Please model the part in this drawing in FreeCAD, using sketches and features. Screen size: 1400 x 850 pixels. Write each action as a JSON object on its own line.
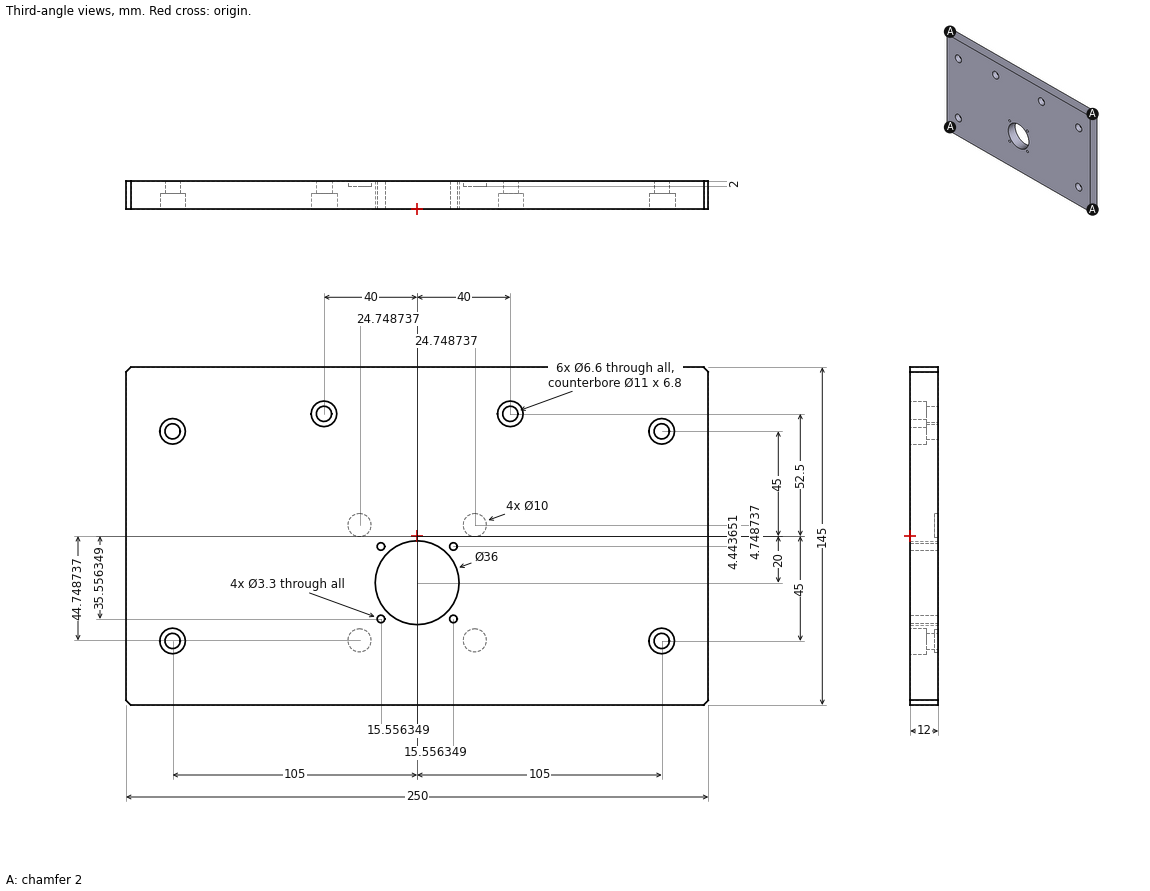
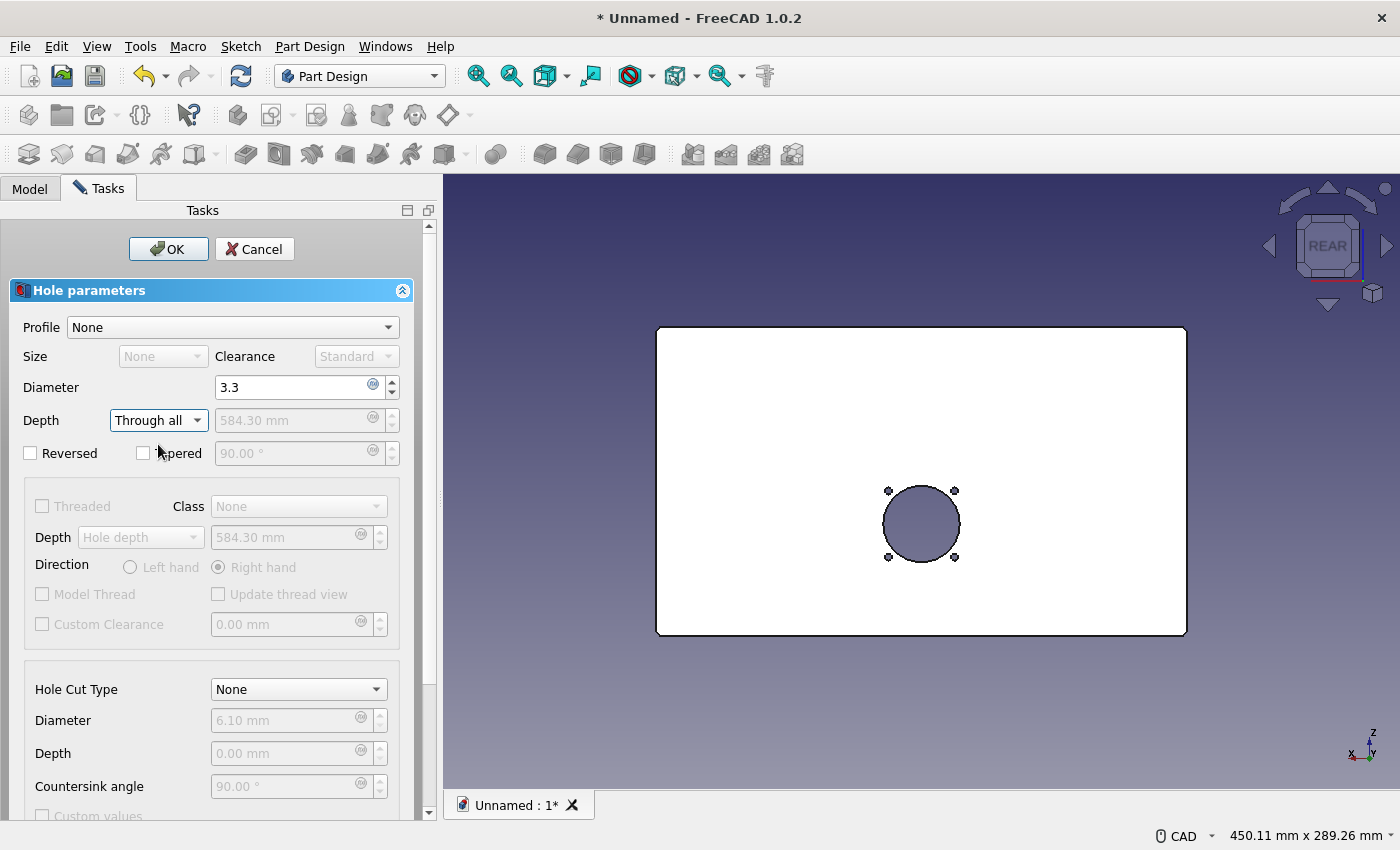
{"action": "left_click", "coordinate": [169, 249]}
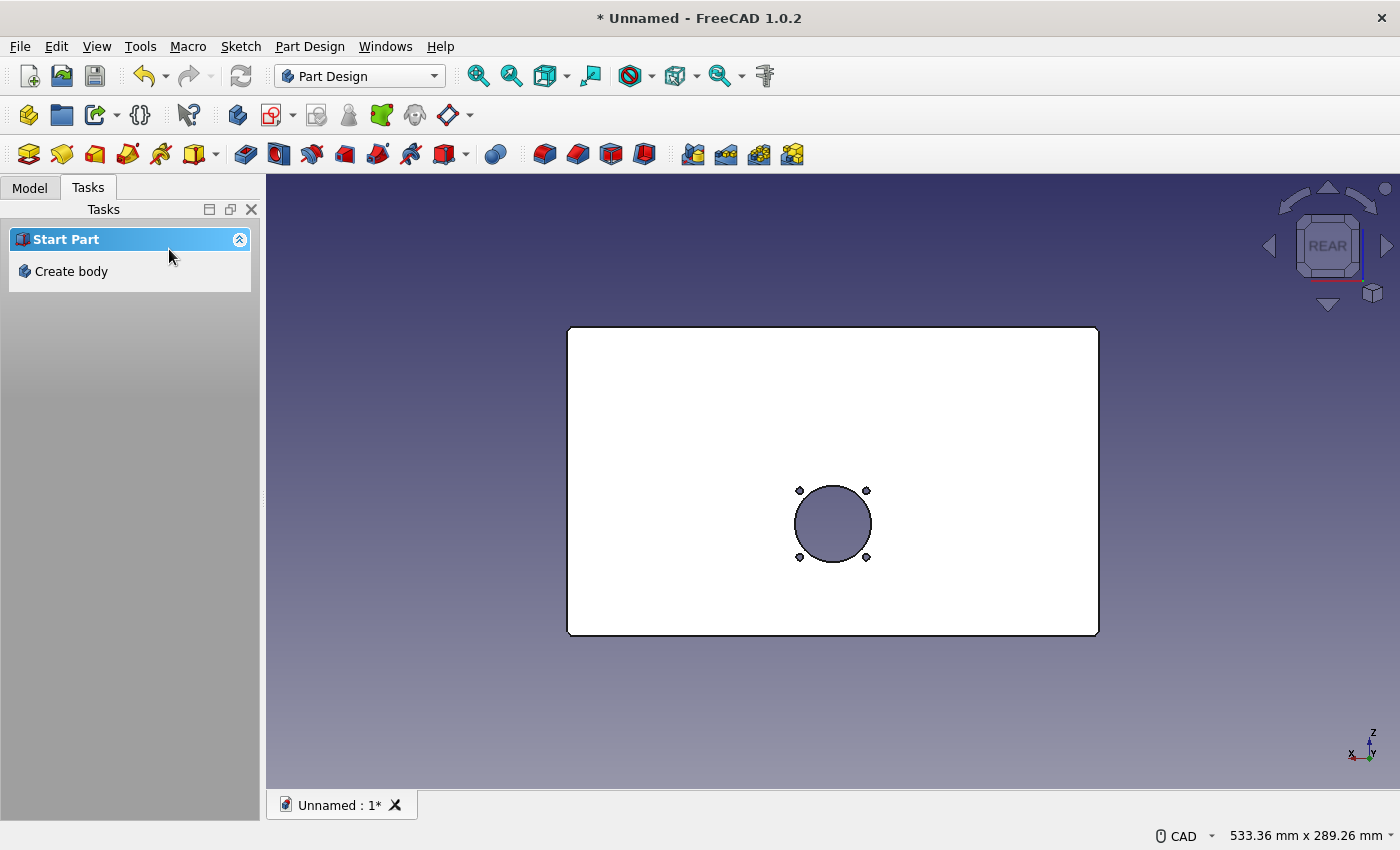
{"action": "left_click", "coordinate": [270, 116]}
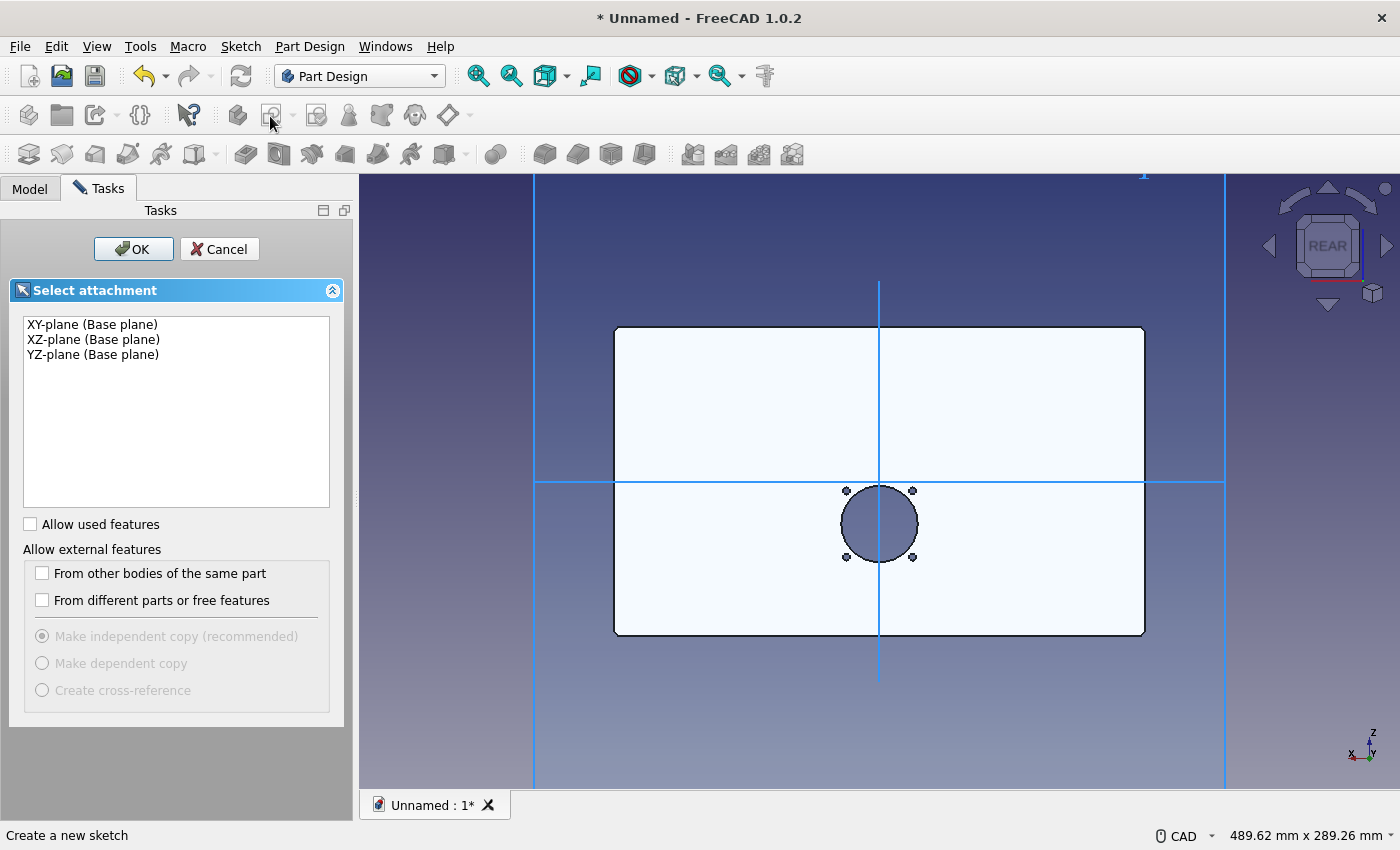
{"action": "left_click", "coordinate": [84, 340]}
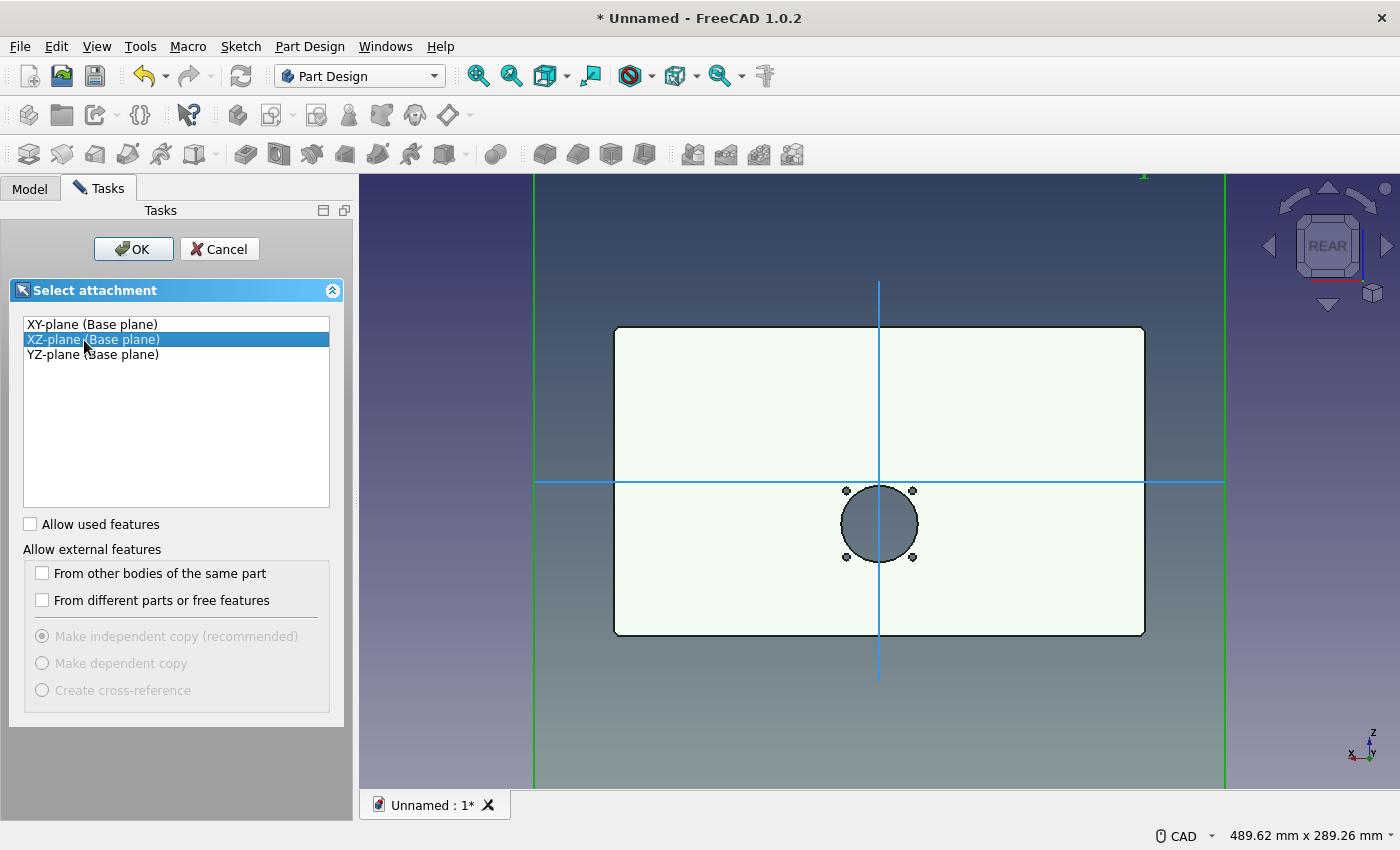
{"action": "left_click", "coordinate": [134, 249]}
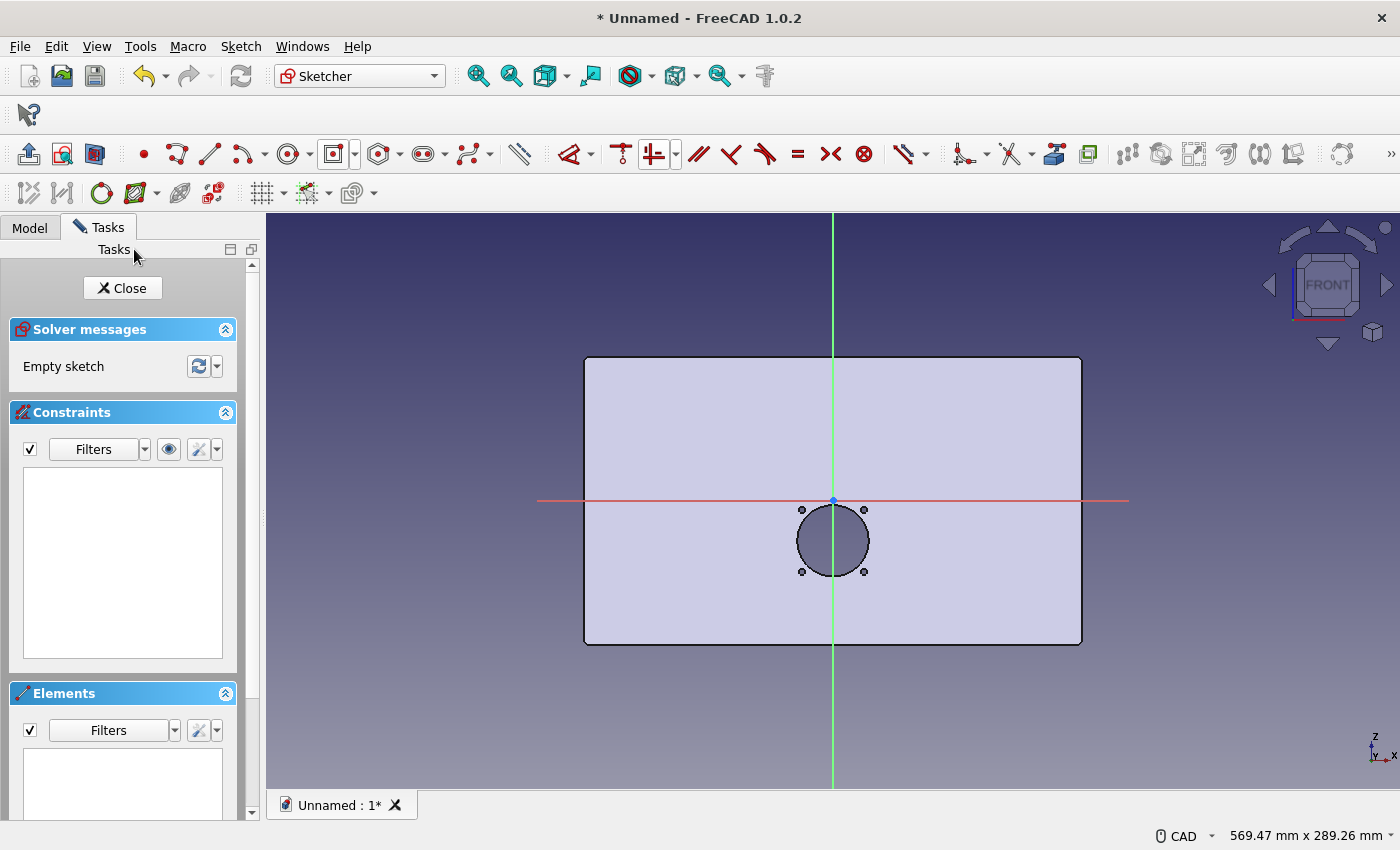
{"action": "scroll", "coordinate": [972, 478], "scroll_direction": "up", "scroll_amount": 2}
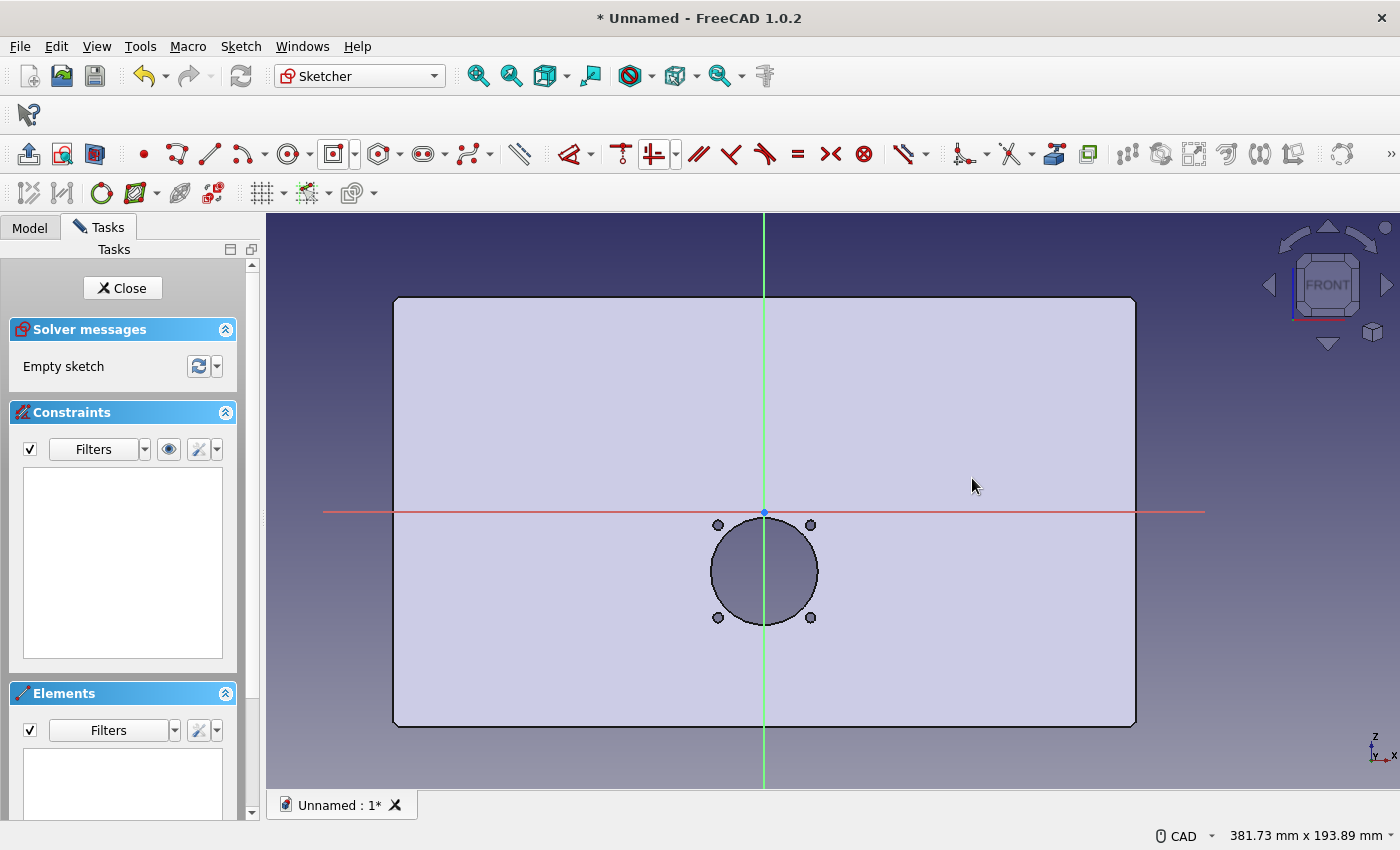
{"action": "key", "text": "g c"}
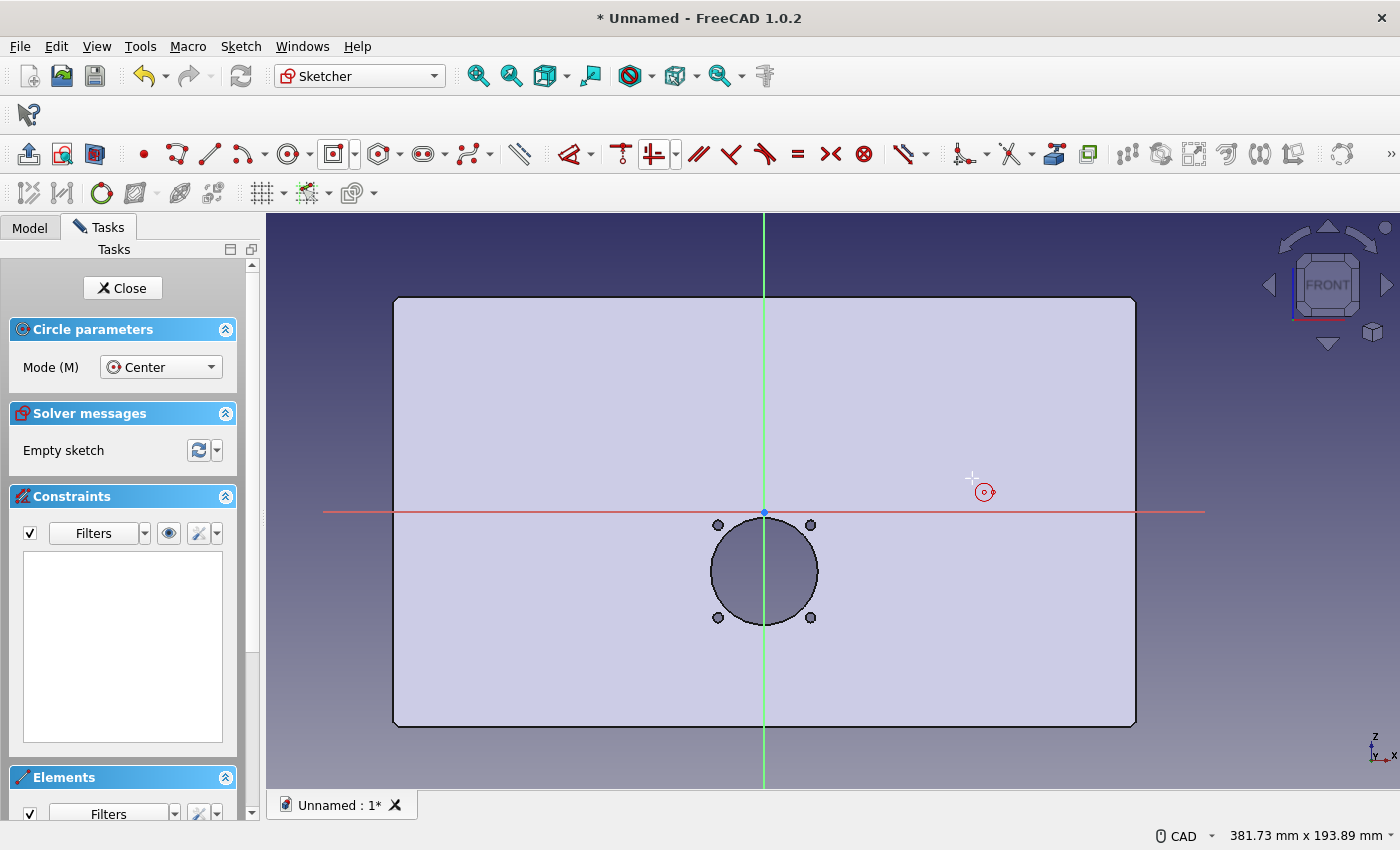
{"action": "scroll", "coordinate": [883, 356], "scroll_direction": "up", "scroll_amount": 5}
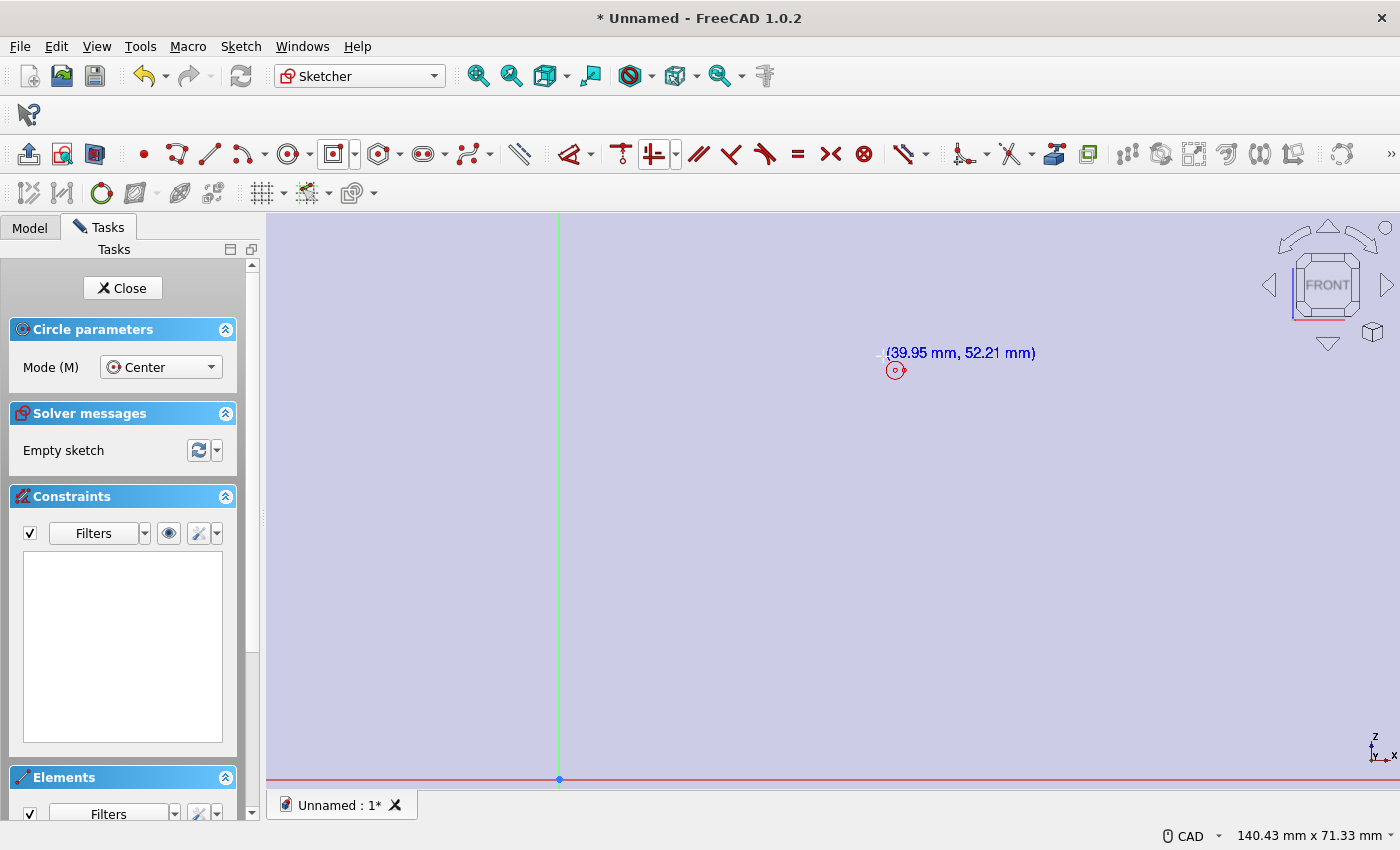
{"action": "left_click", "coordinate": [882, 356]}
{"action": "mouse_move", "coordinate": [901, 337]}